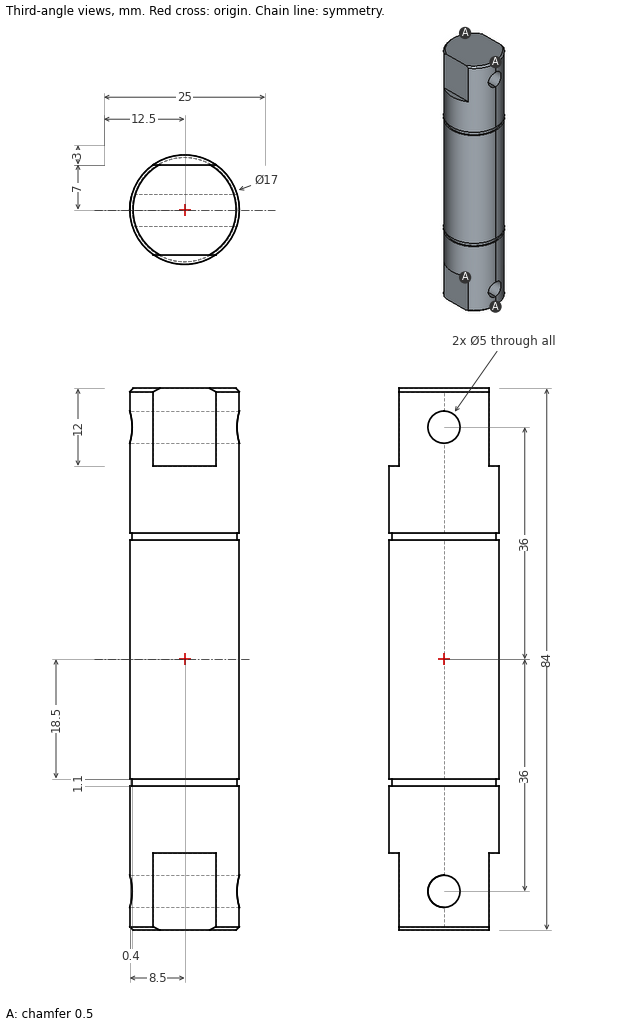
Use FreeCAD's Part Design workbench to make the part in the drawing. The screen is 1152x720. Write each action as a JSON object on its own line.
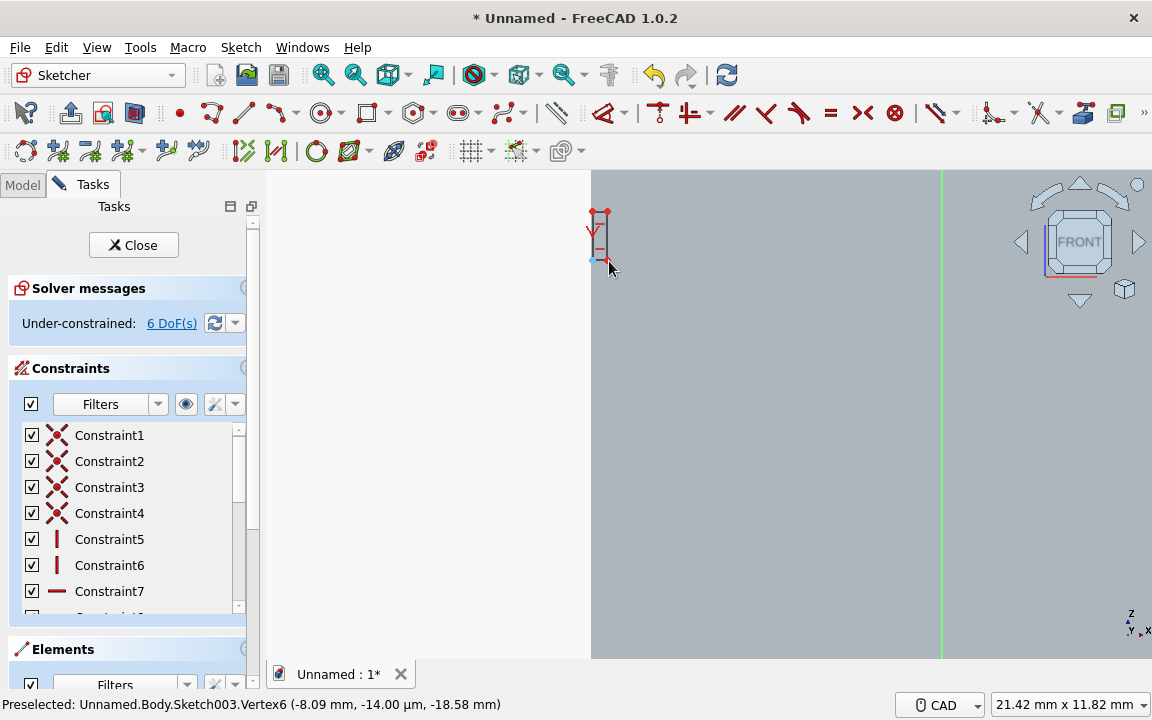
{"action": "left_click", "coordinate": [607, 260]}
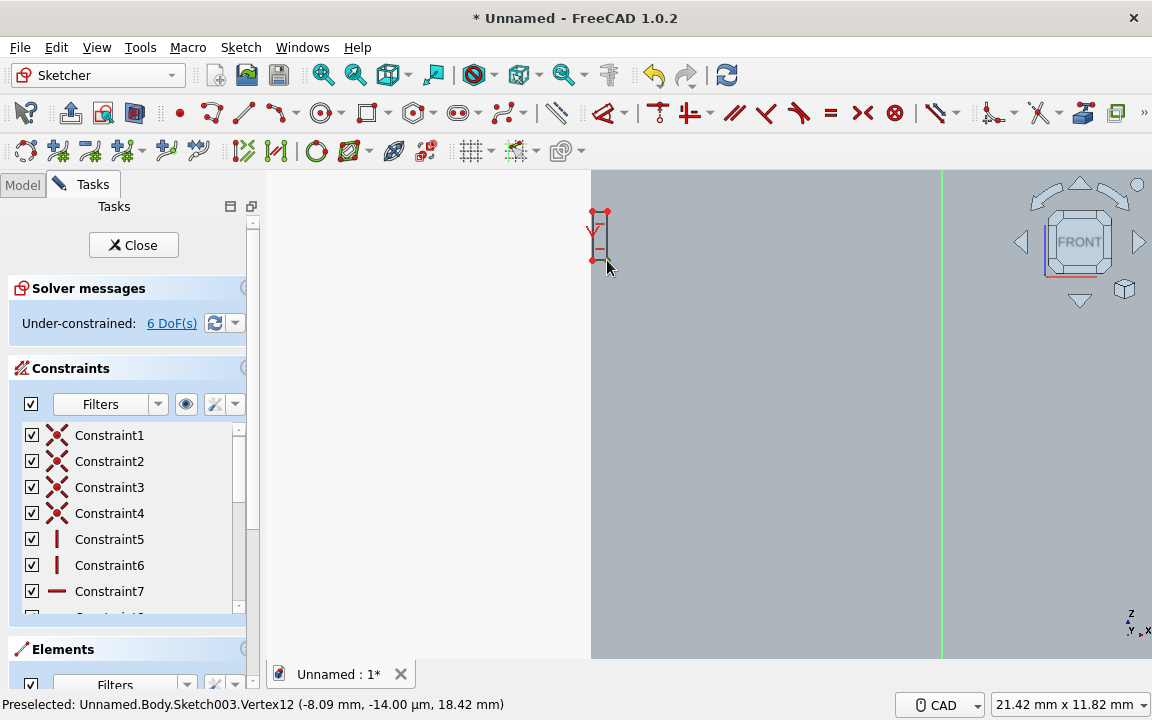
{"action": "scroll", "coordinate": [609, 261], "scroll_direction": "down", "scroll_amount": 8}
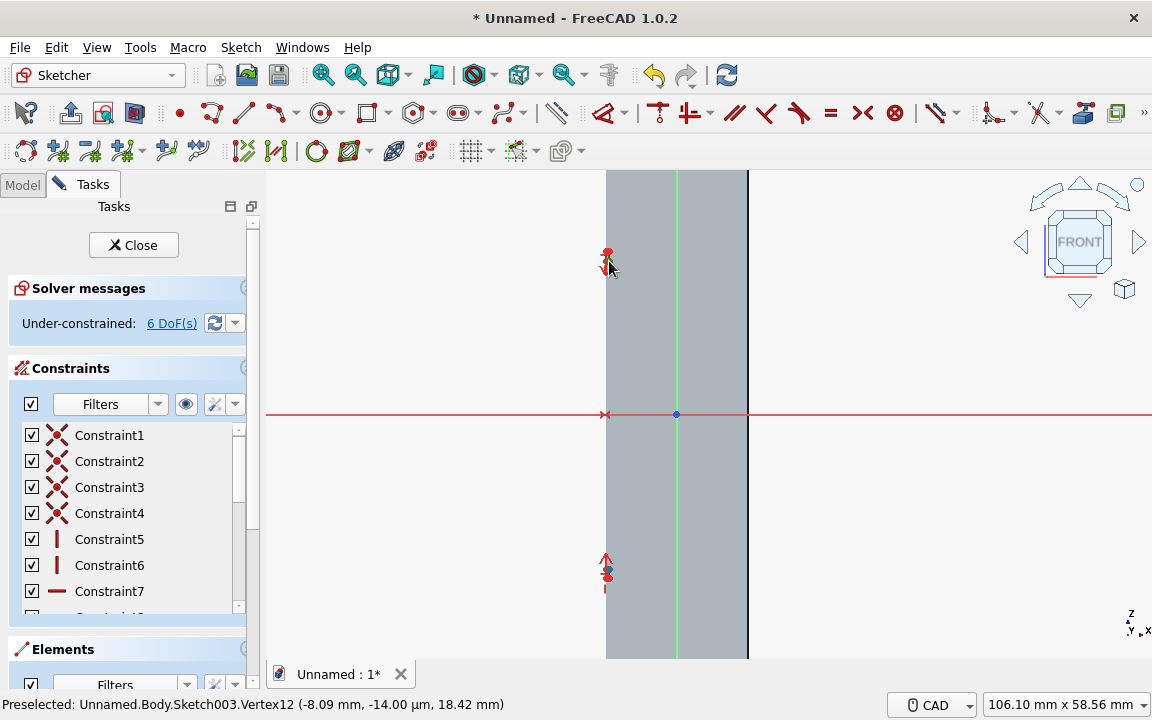
{"action": "left_click", "coordinate": [344, 415]}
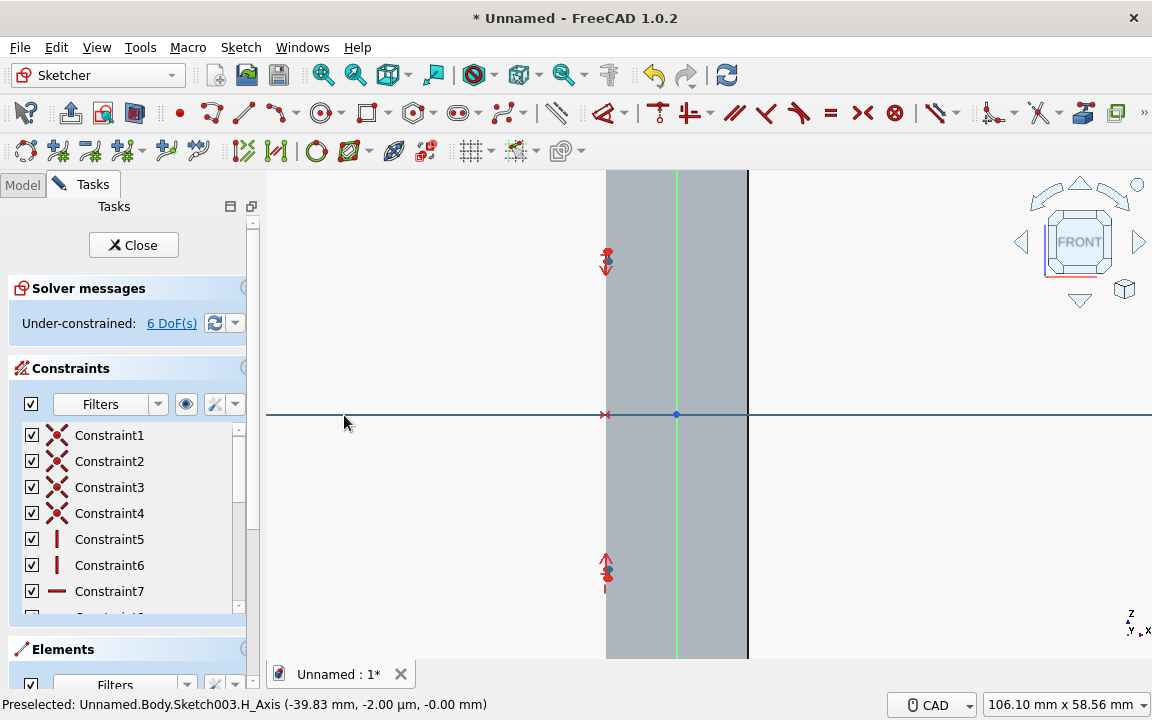
{"action": "left_click", "coordinate": [864, 114]}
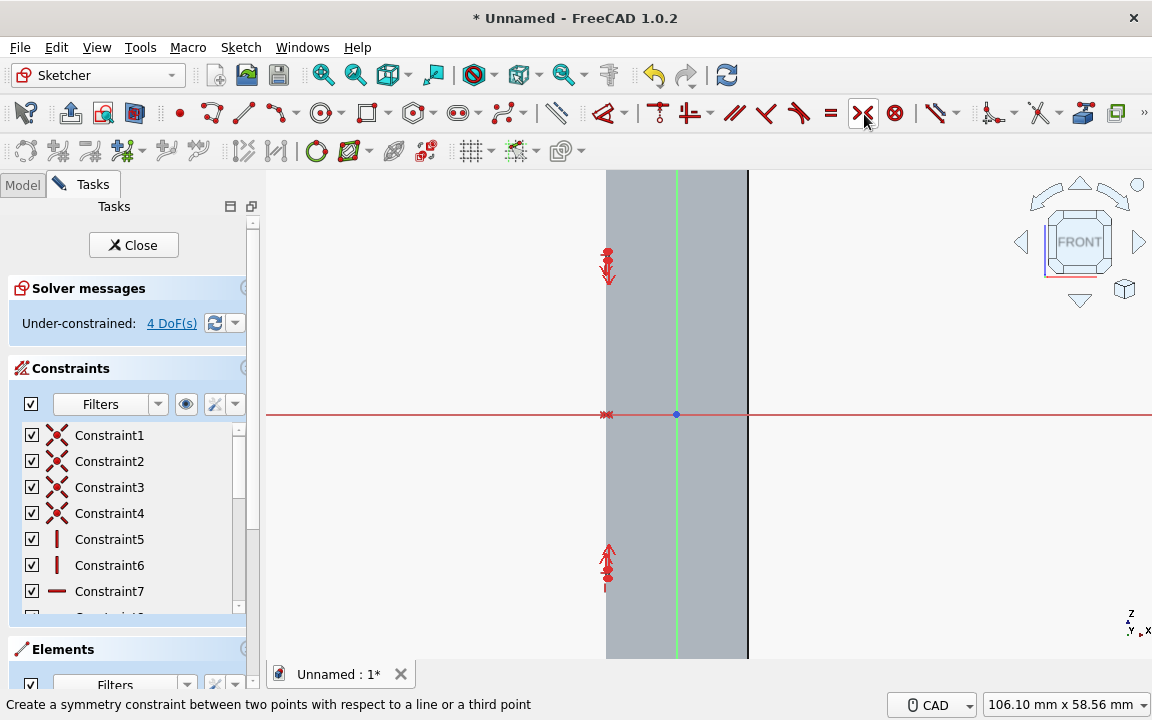
{"action": "left_click", "coordinate": [604, 114]}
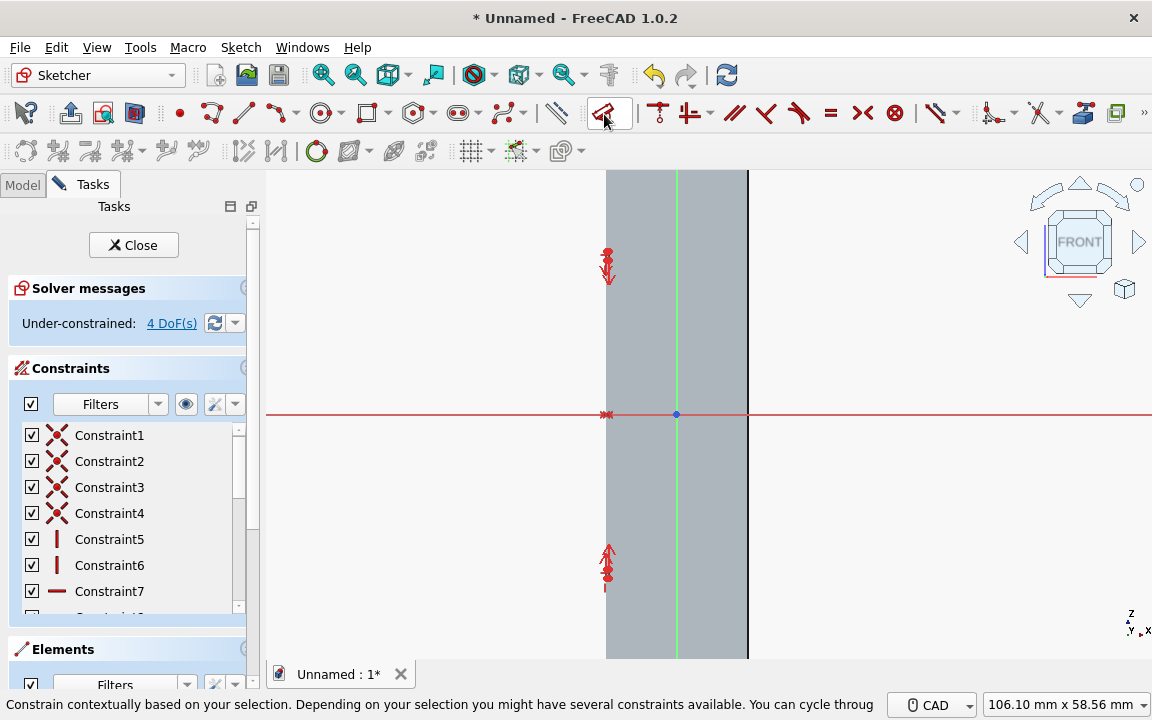
{"action": "scroll", "coordinate": [606, 573], "scroll_direction": "up", "scroll_amount": 8}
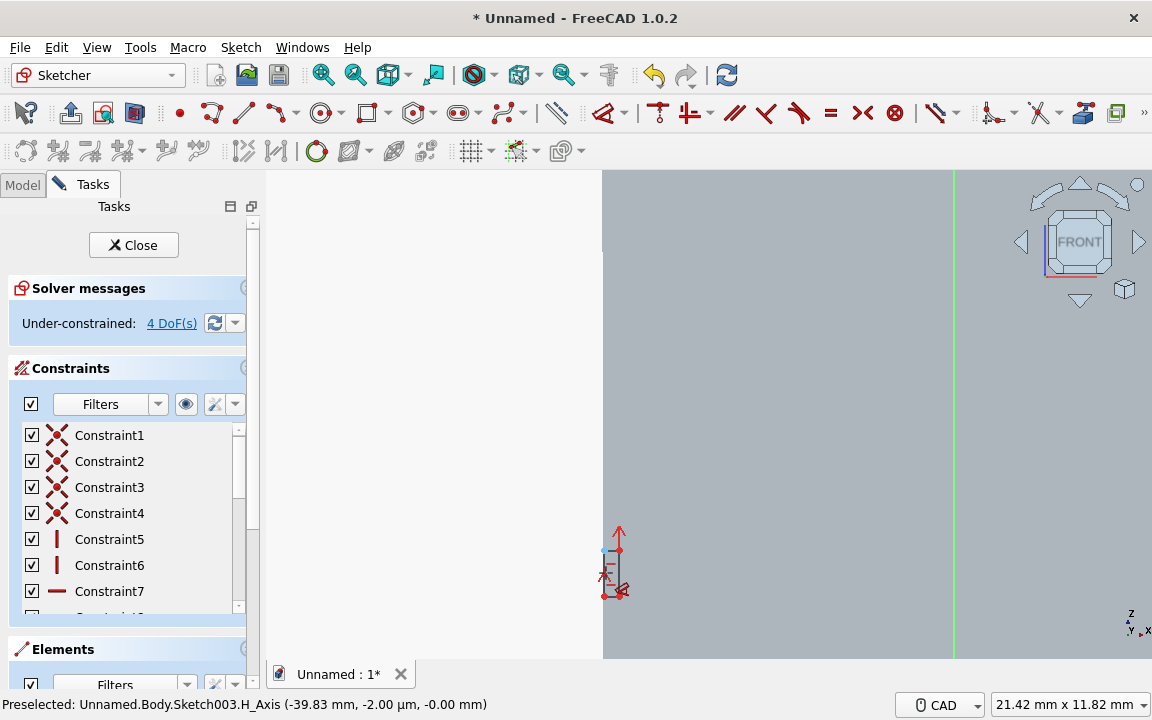
{"action": "left_click", "coordinate": [604, 569]}
{"action": "left_click", "coordinate": [570, 574]}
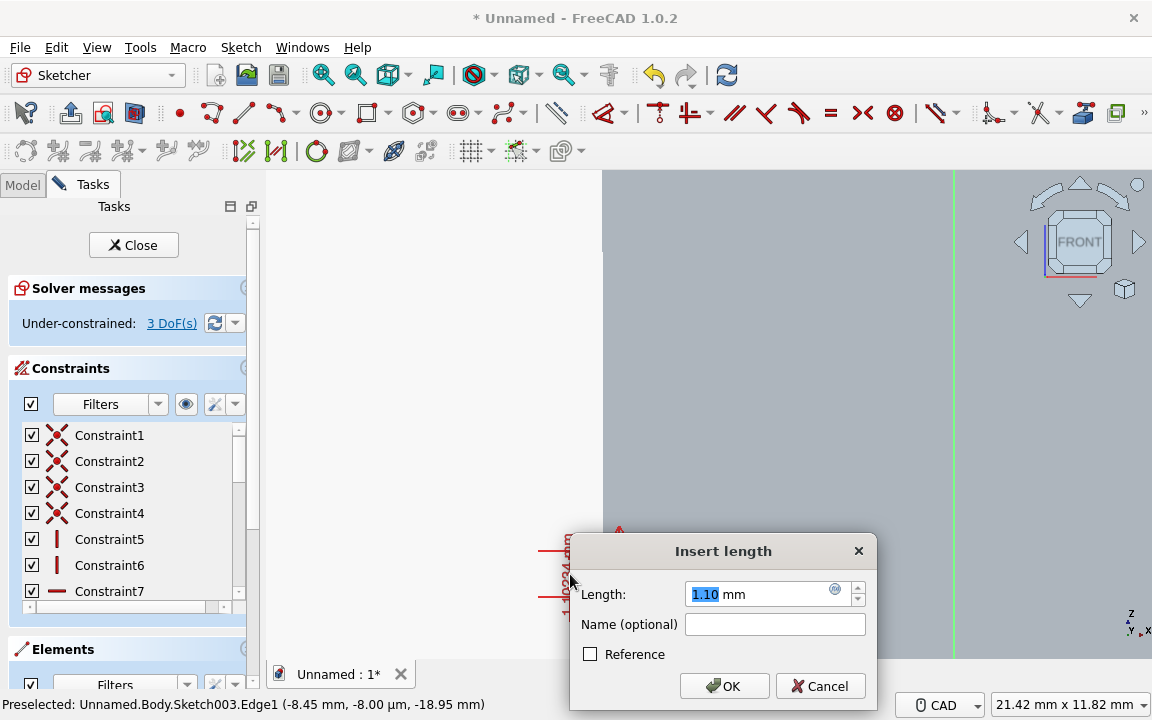
{"action": "type", "text": "1.1"}
{"action": "key", "text": "Return"}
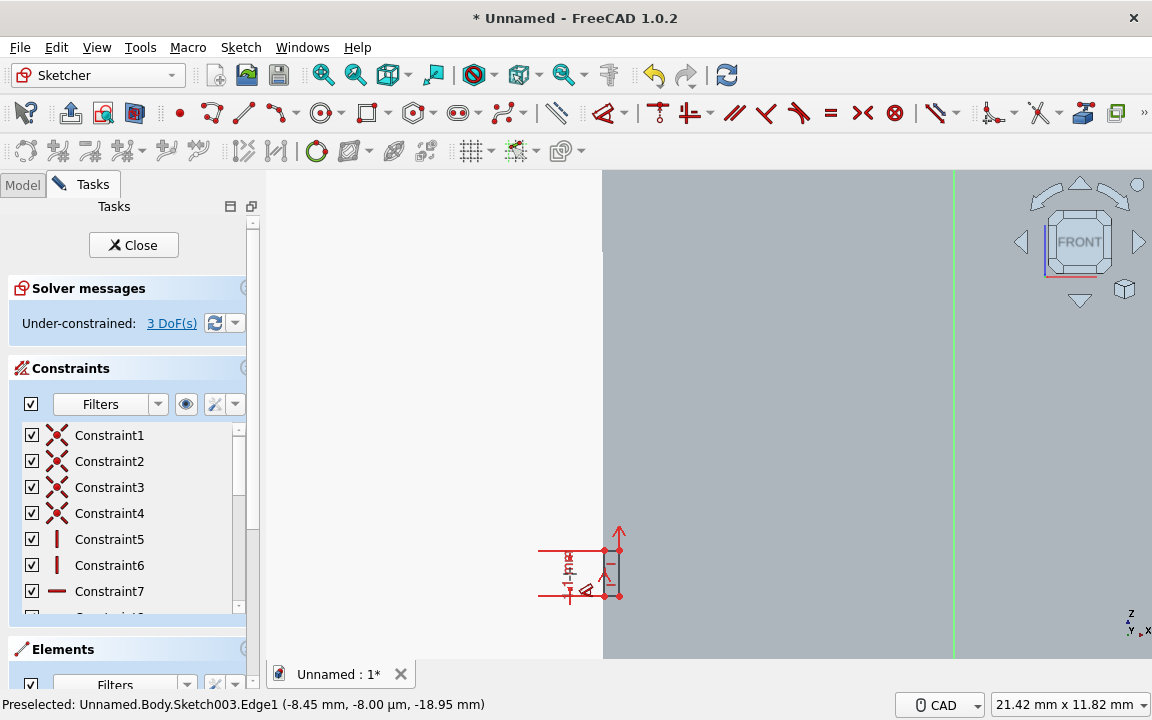
{"action": "scroll", "coordinate": [612, 596], "scroll_direction": "up", "scroll_amount": 5}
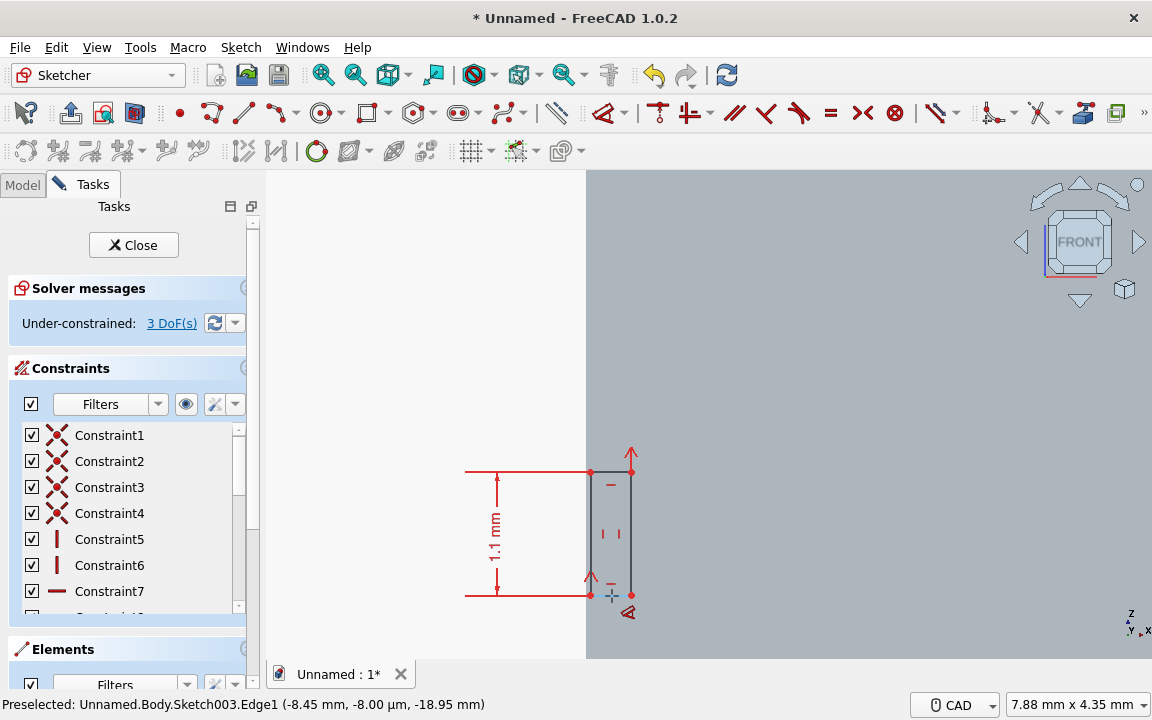
{"action": "left_click", "coordinate": [611, 596]}
{"action": "left_click", "coordinate": [611, 630]}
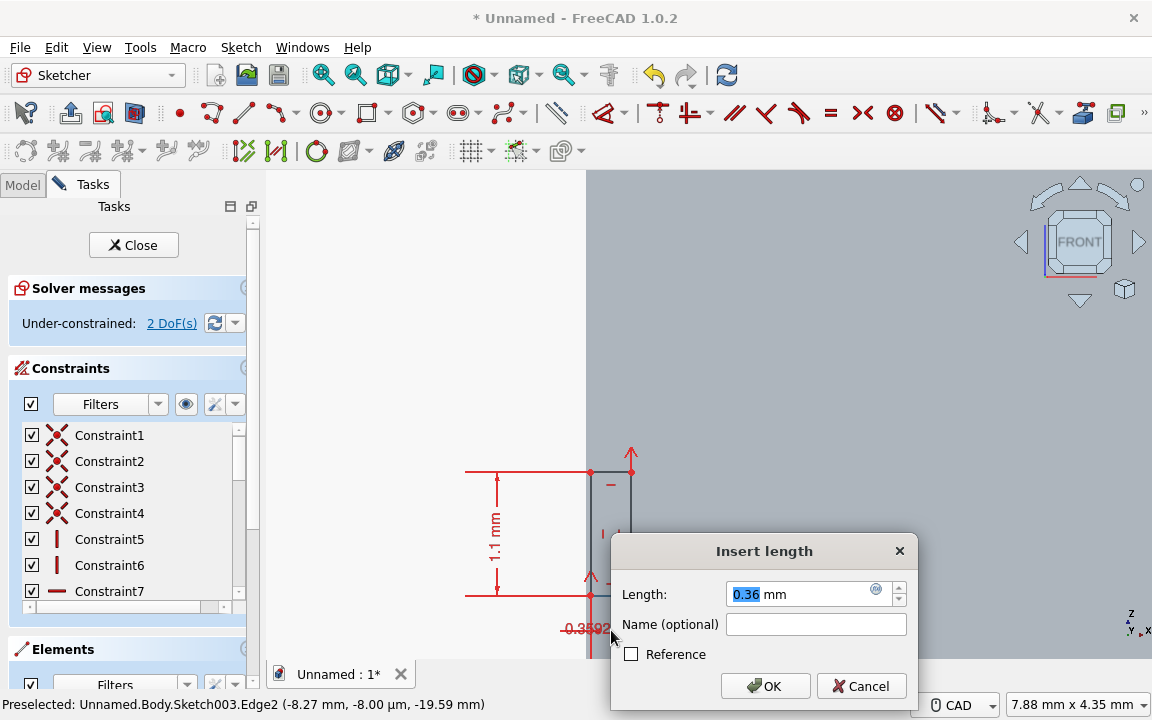
{"action": "type", "text": "0.4"}
{"action": "key", "text": "Return"}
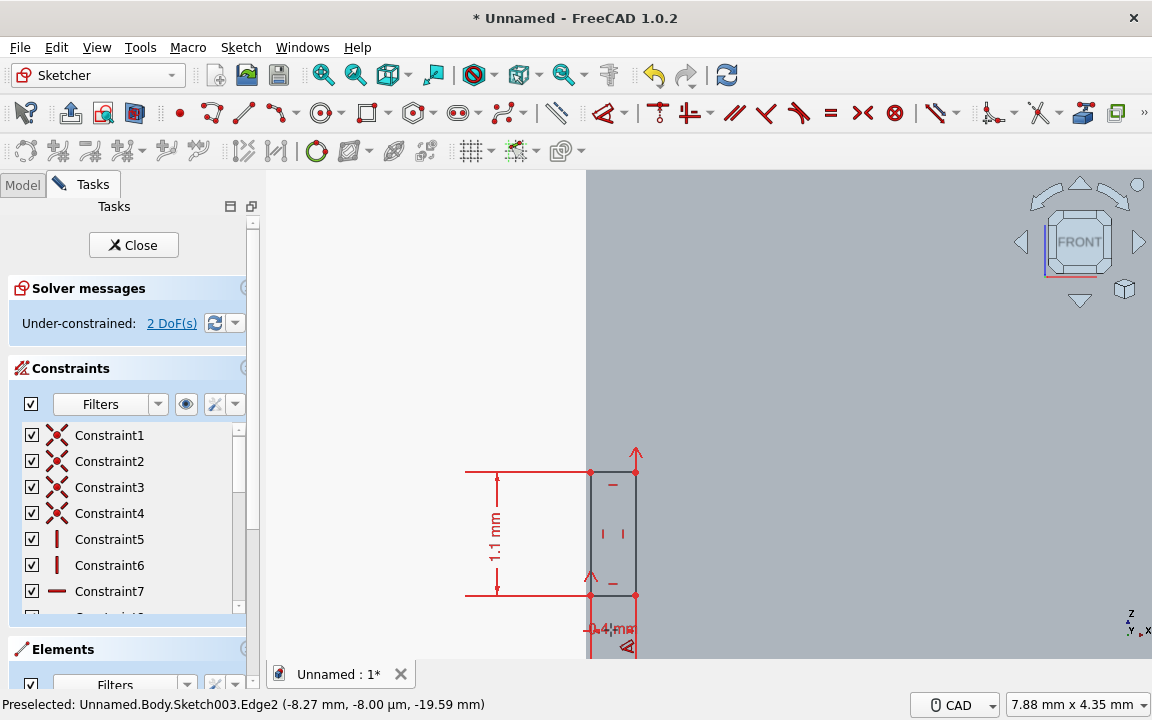
{"action": "scroll", "coordinate": [607, 577], "scroll_direction": "down", "scroll_amount": 13}